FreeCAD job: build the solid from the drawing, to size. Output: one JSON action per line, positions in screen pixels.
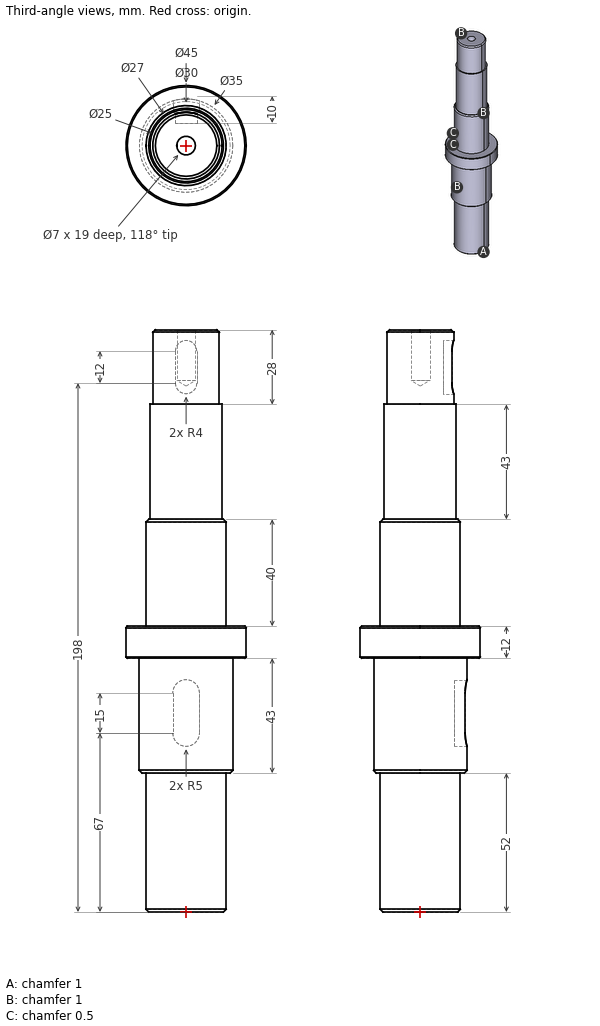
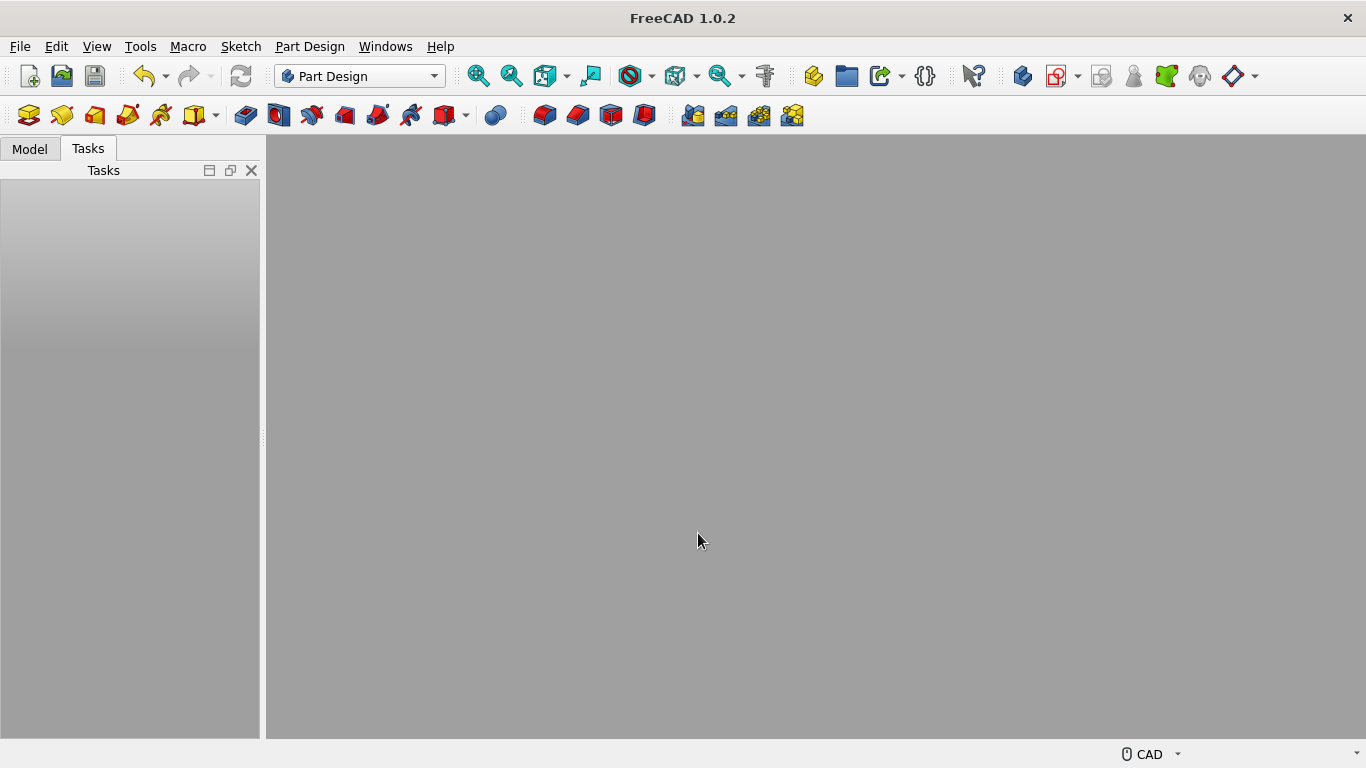
{"action": "key", "text": "ctrl+n"}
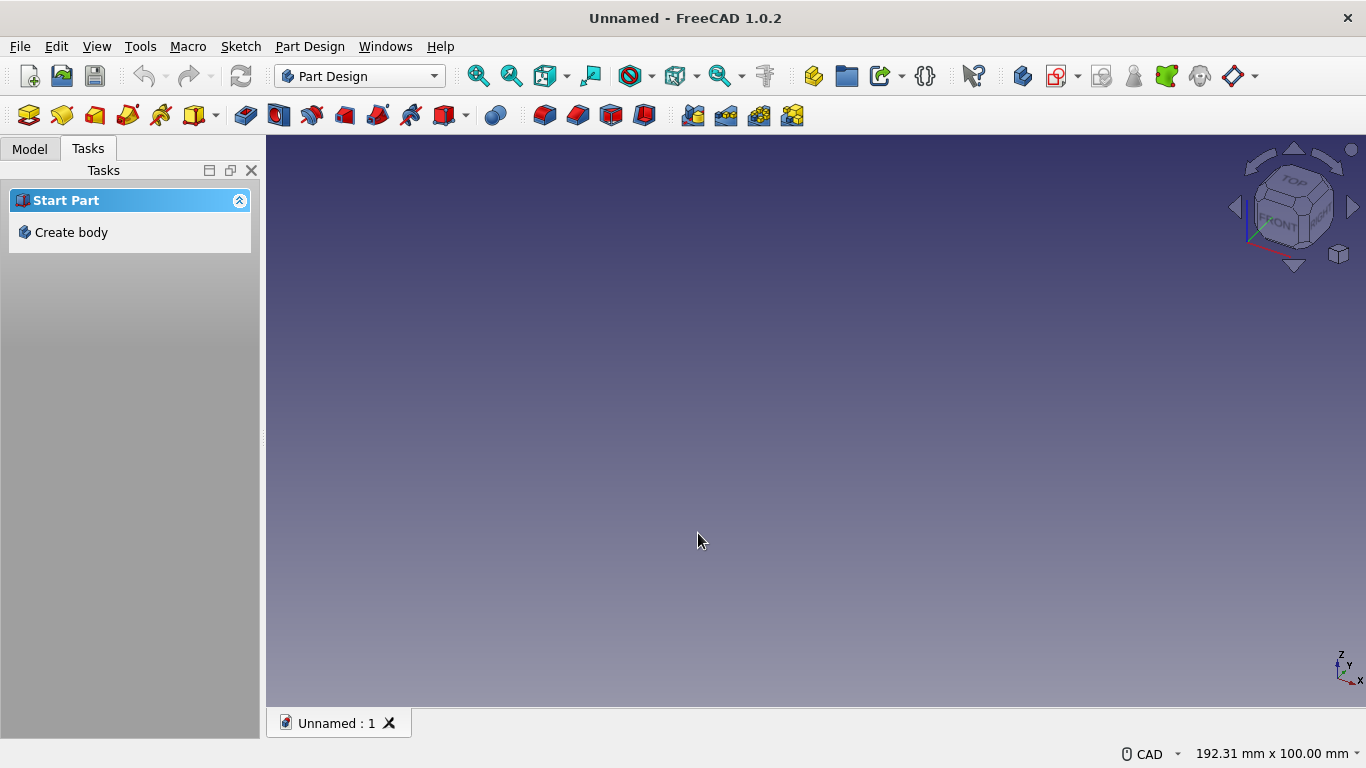
{"action": "left_click", "coordinate": [1056, 76]}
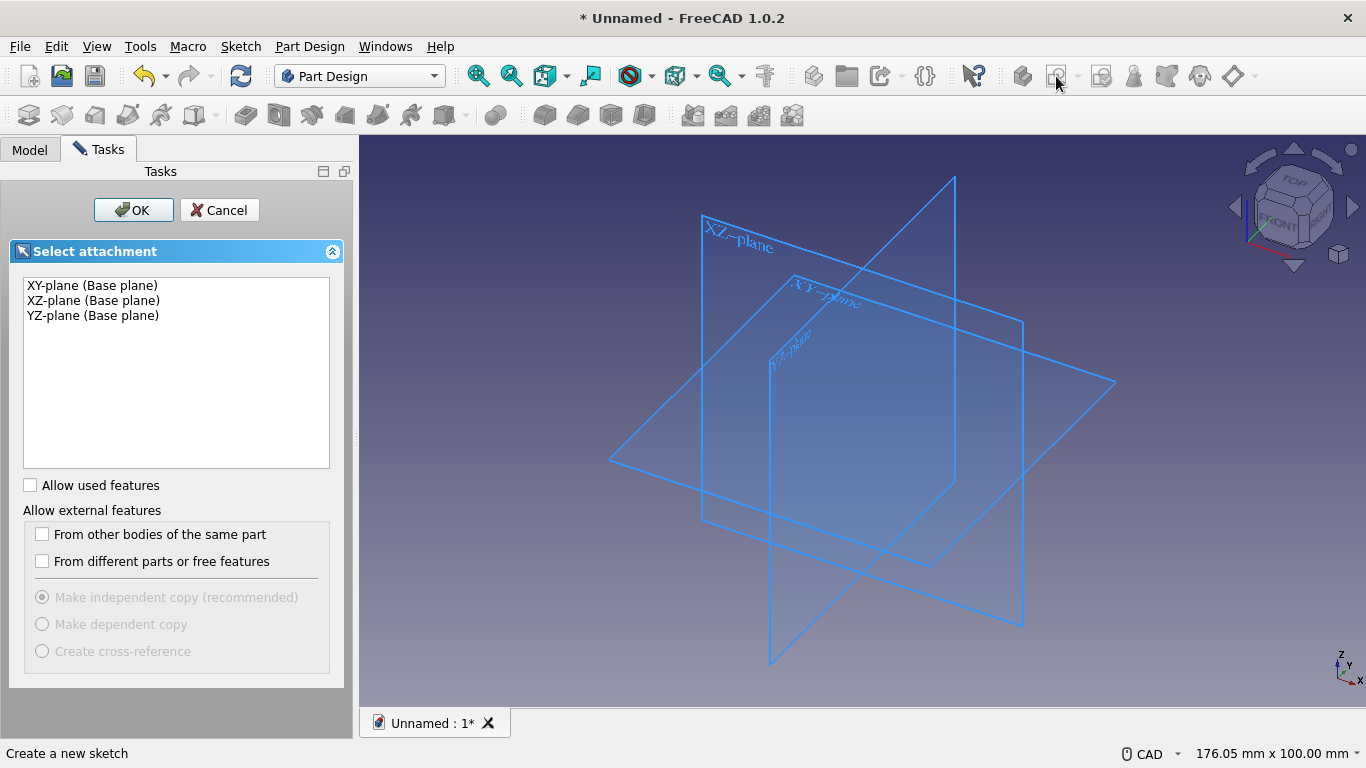
{"action": "left_click", "coordinate": [84, 286]}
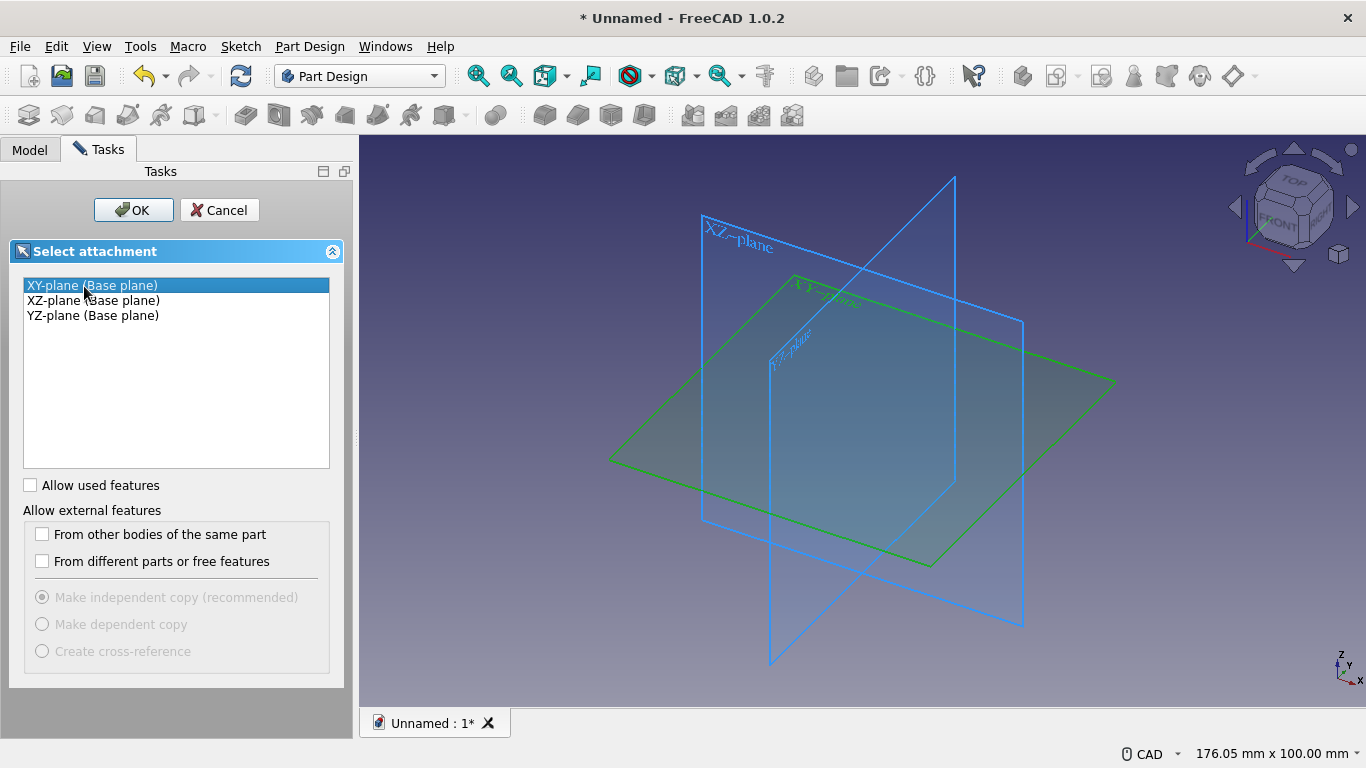
{"action": "left_click", "coordinate": [134, 210]}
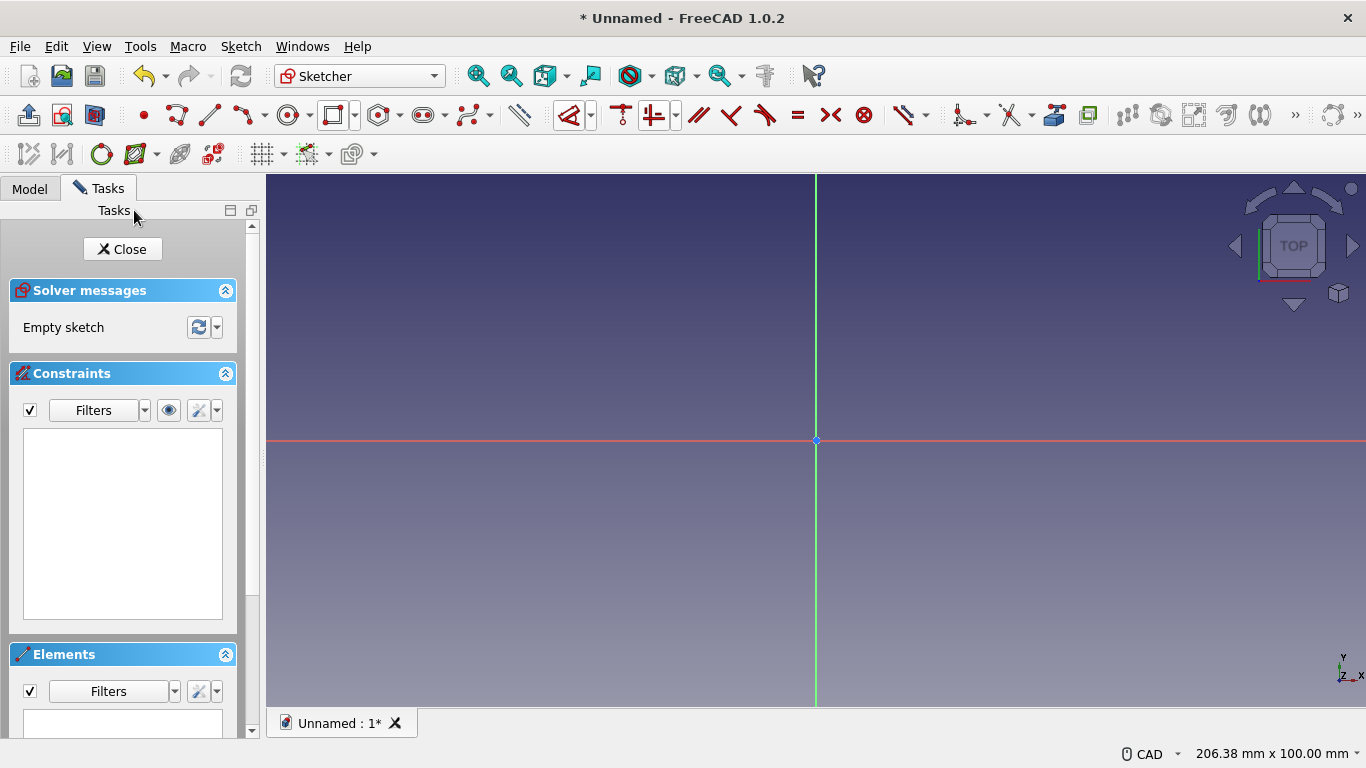
{"action": "scroll", "coordinate": [872, 440], "scroll_direction": "up", "scroll_amount": 4}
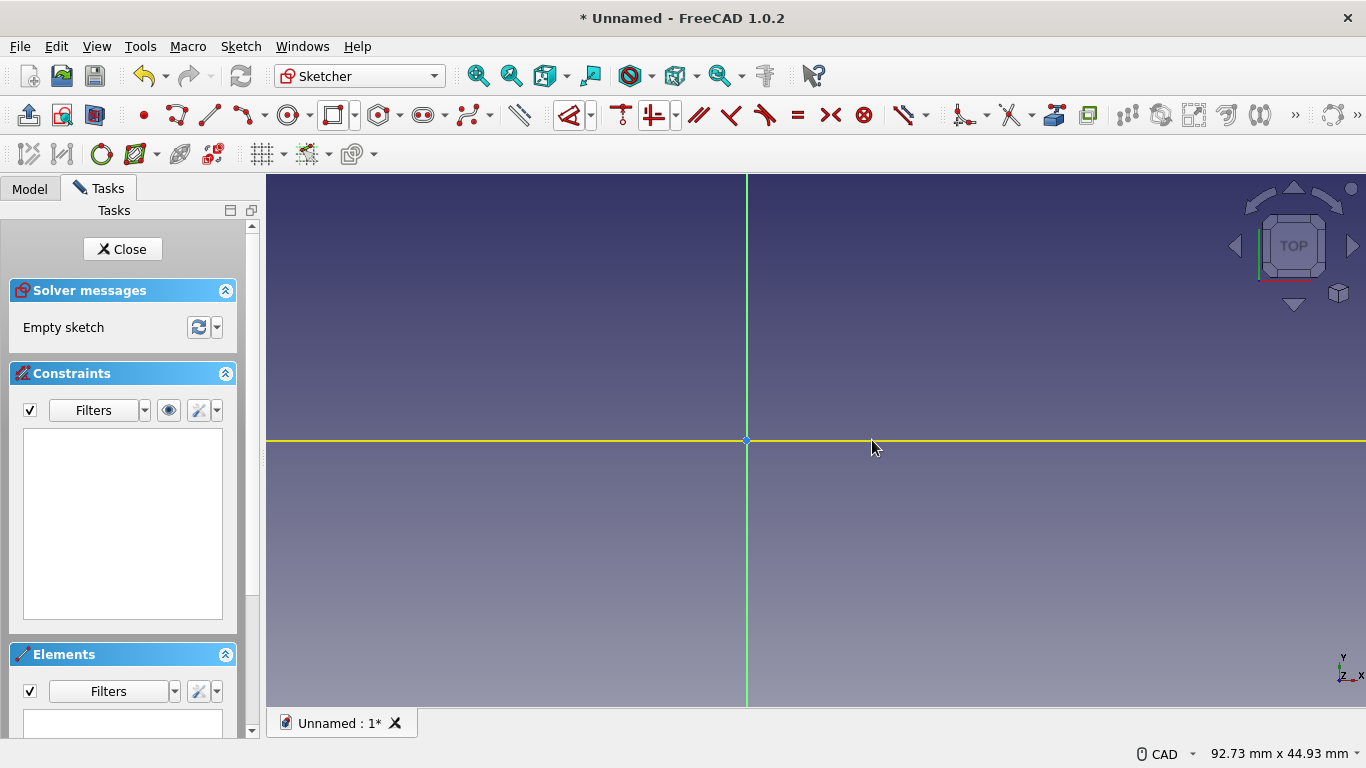
{"action": "key", "text": "g c"}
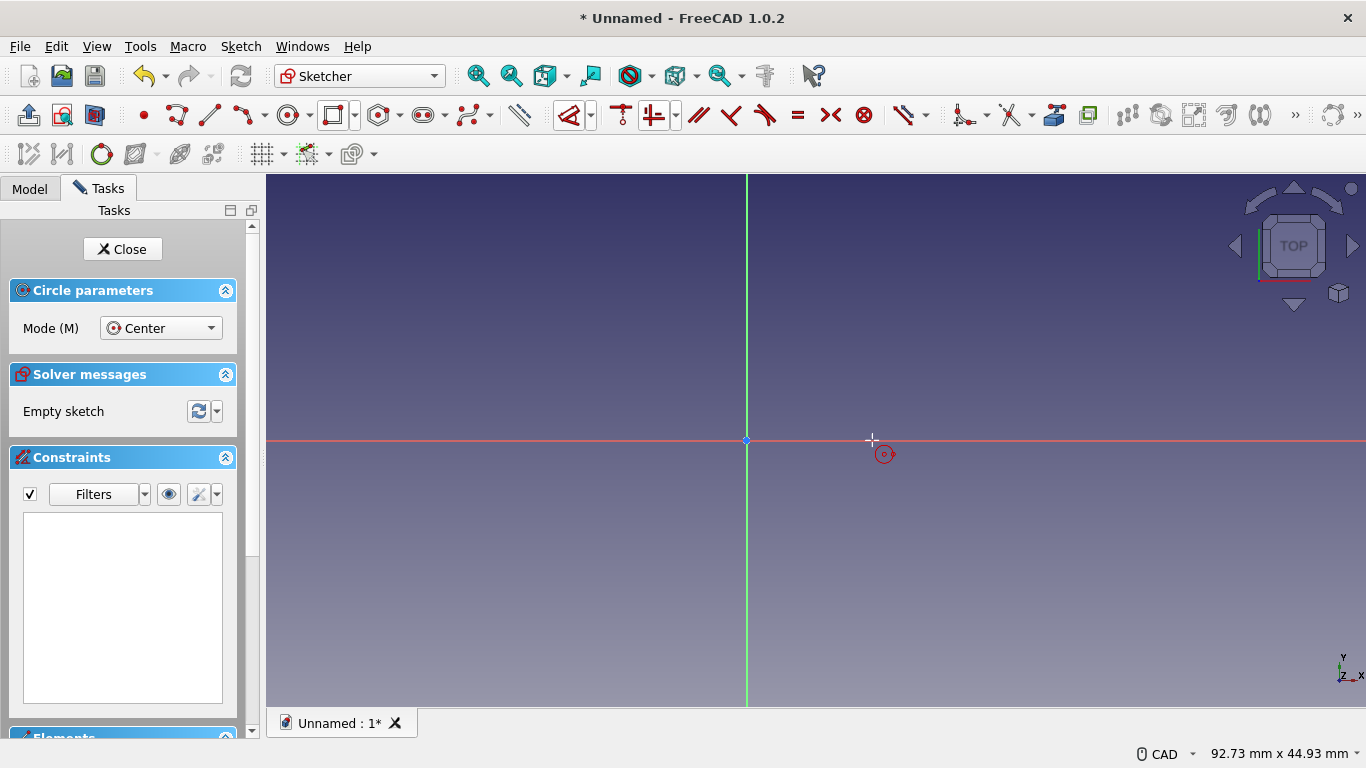
{"action": "left_click", "coordinate": [747, 440]}
{"action": "mouse_move", "coordinate": [873, 315]}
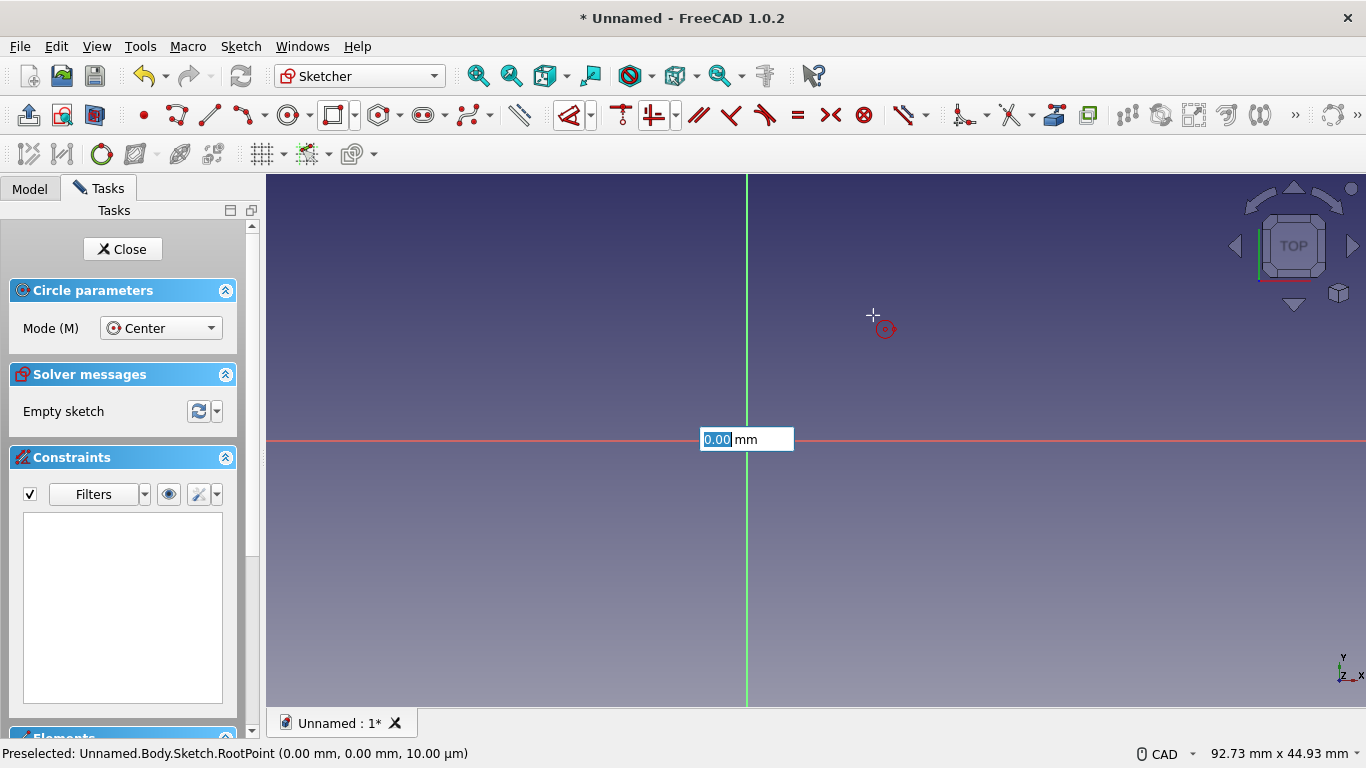
{"action": "type", "text": "30"}
{"action": "key", "text": "Return"}
{"action": "key", "text": "Escape"}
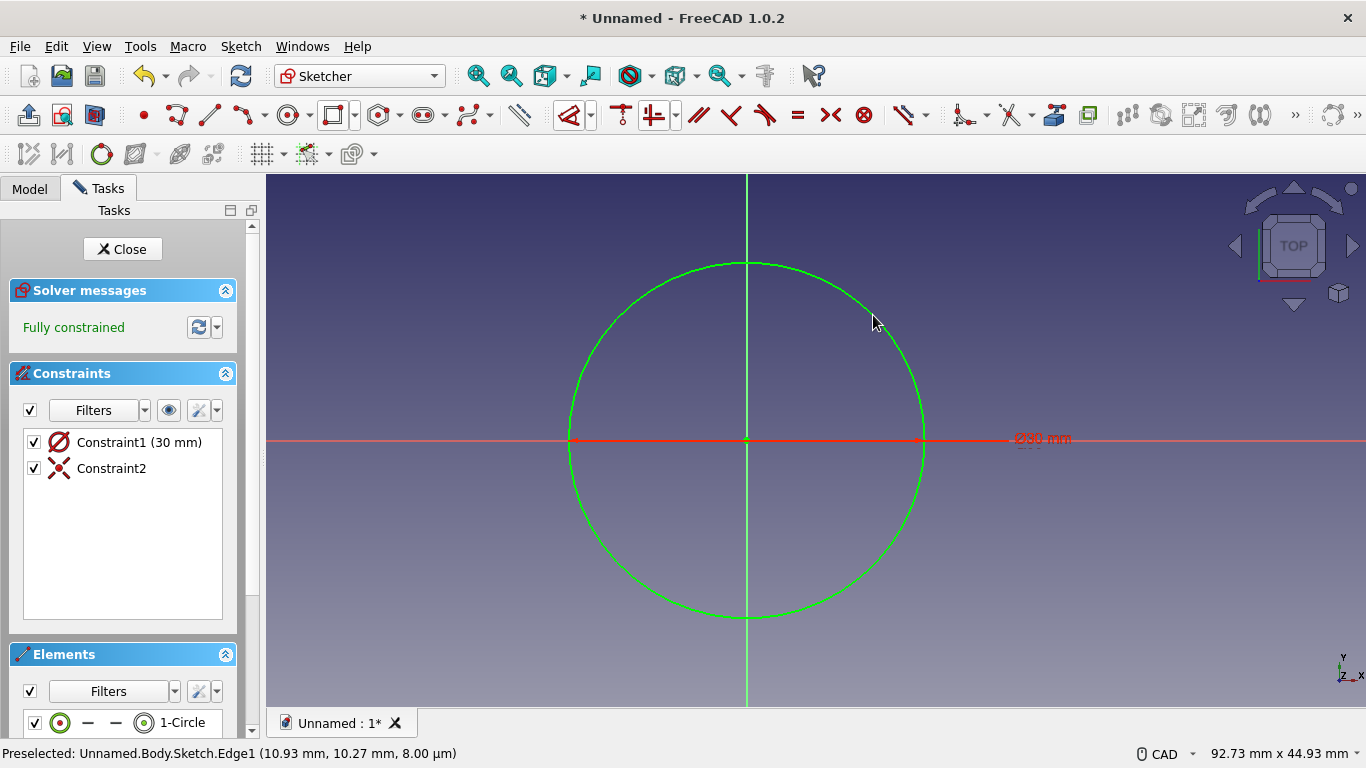
{"action": "left_click", "coordinate": [123, 249]}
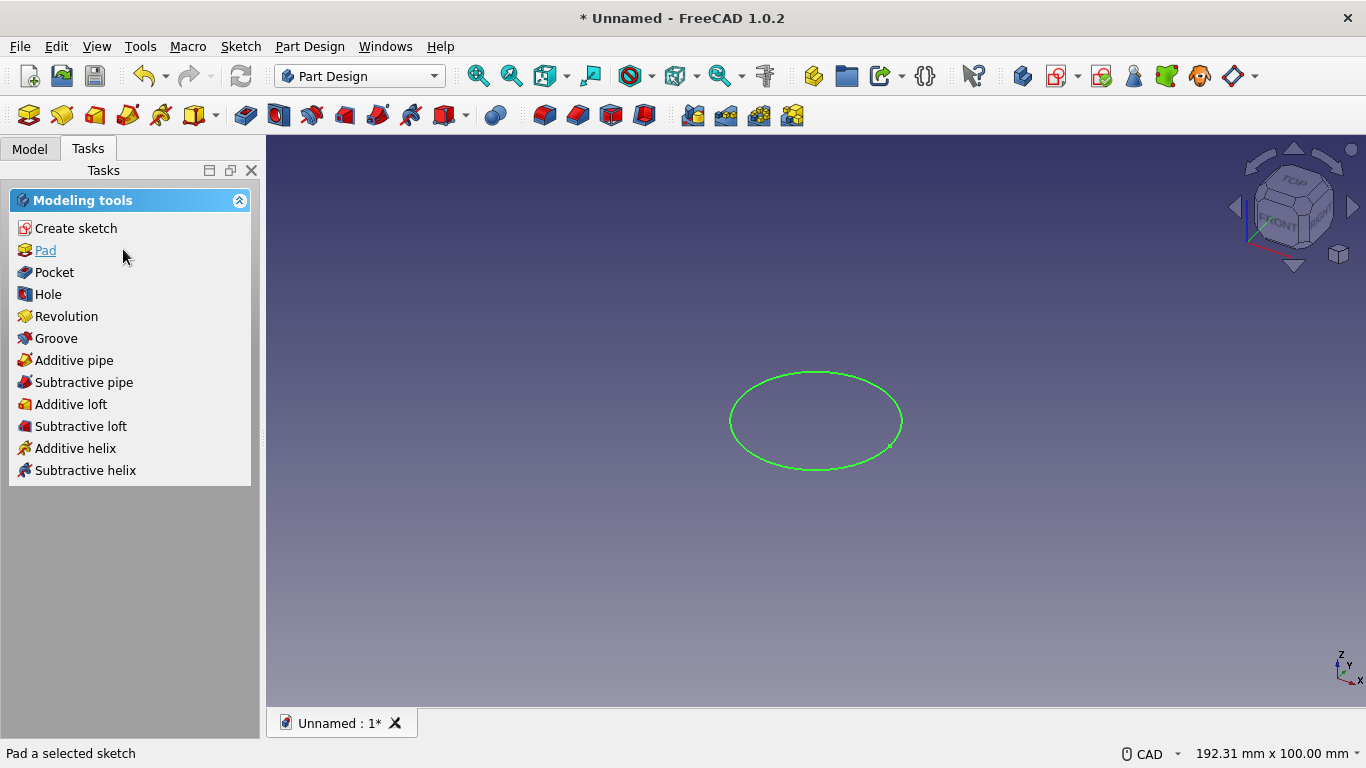
{"action": "left_click", "coordinate": [29, 116]}